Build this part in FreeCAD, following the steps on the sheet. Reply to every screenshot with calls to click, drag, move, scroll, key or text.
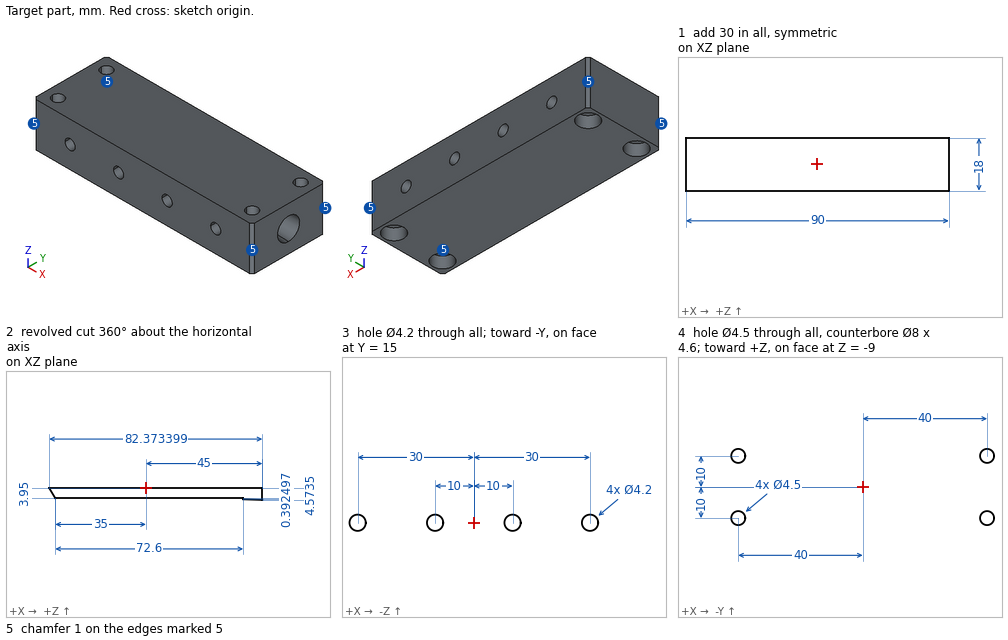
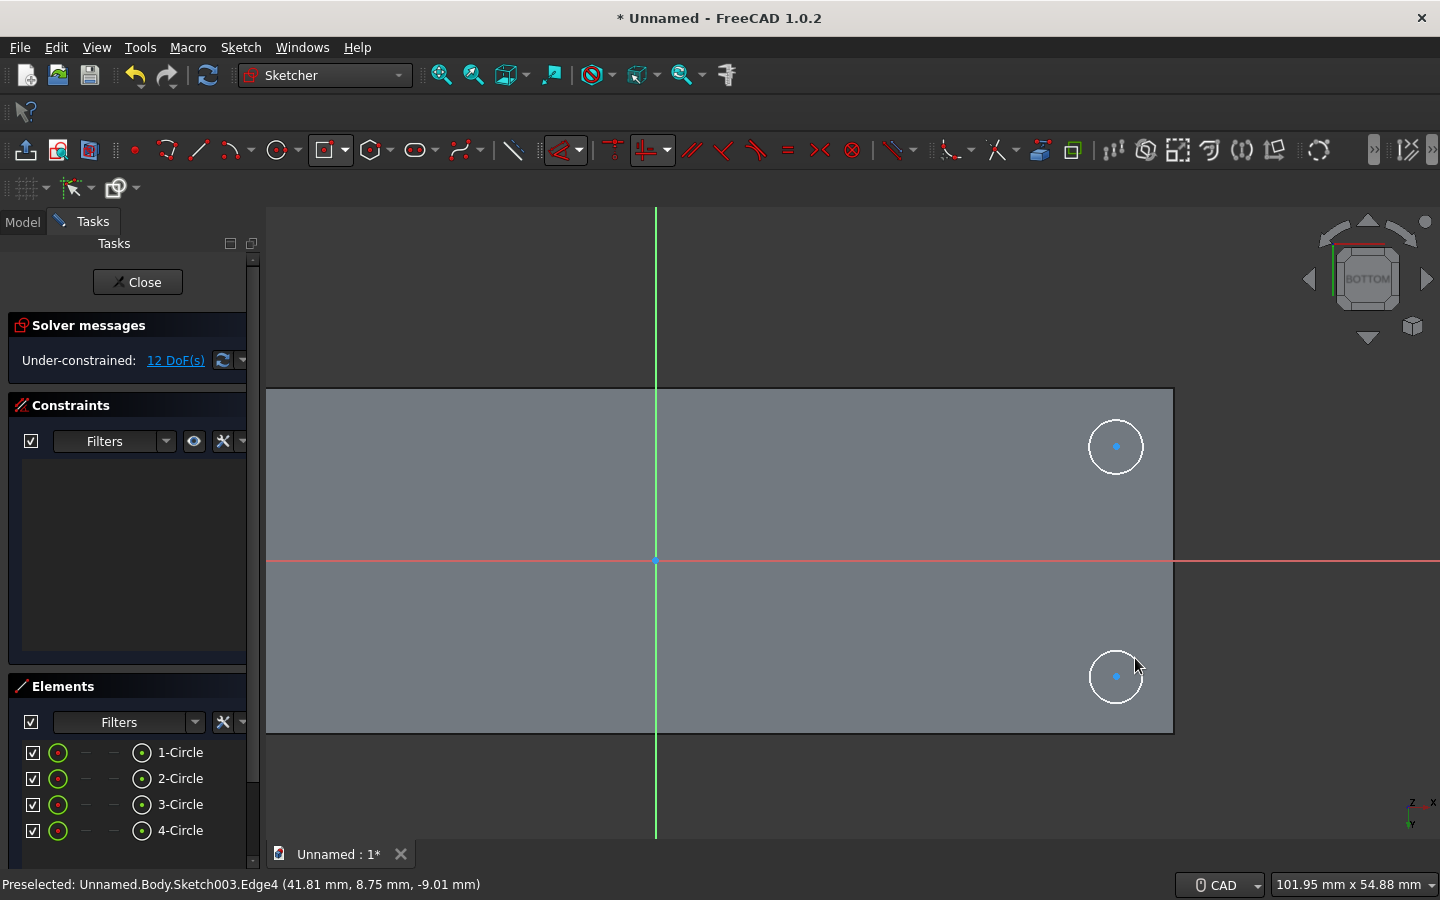
scroll(1046, 446, down, 2)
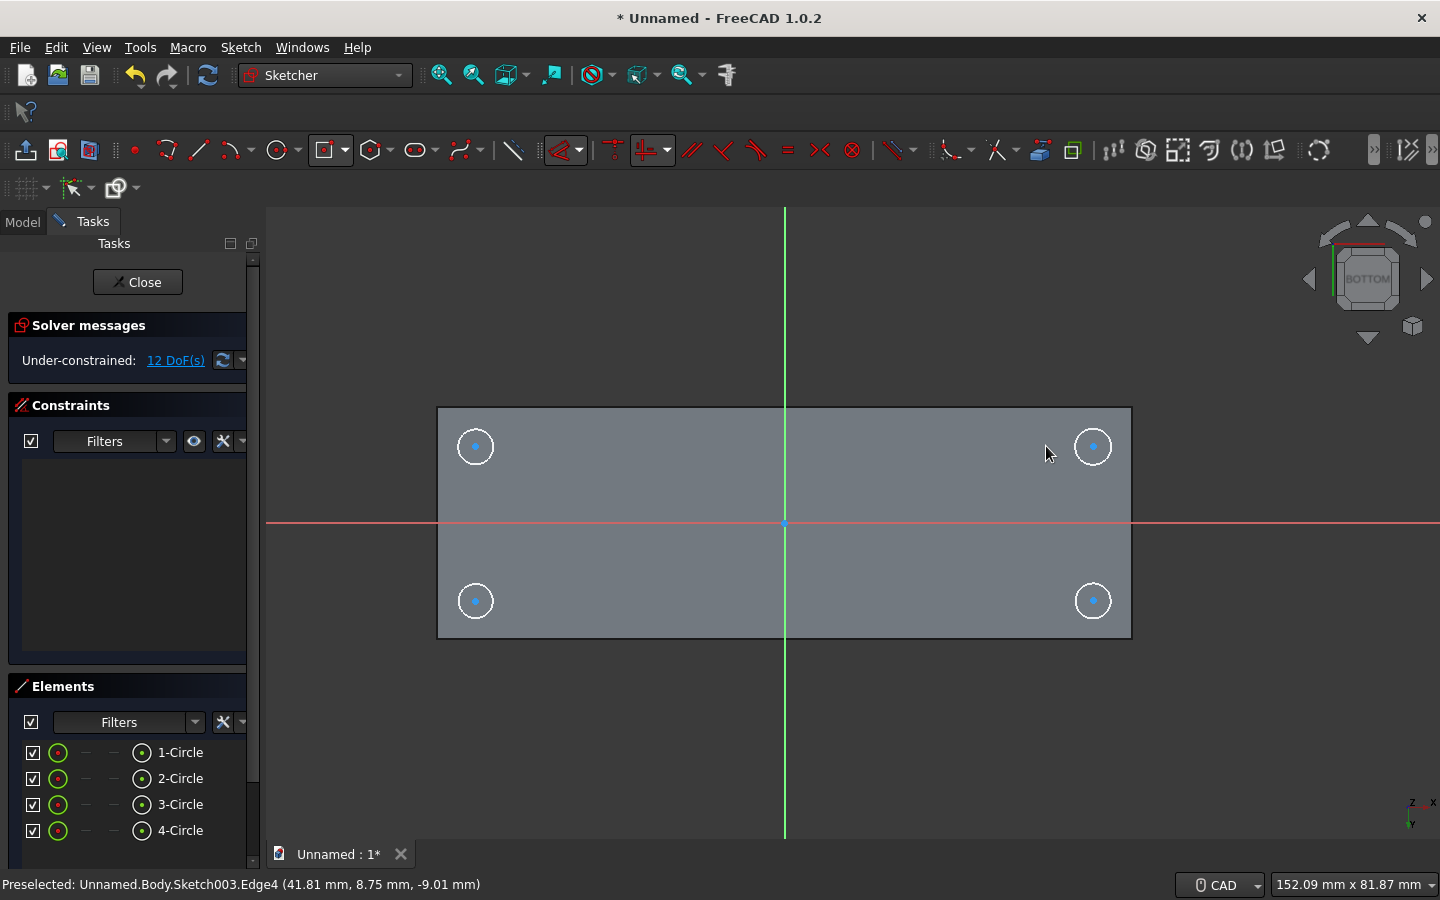
click(488, 589)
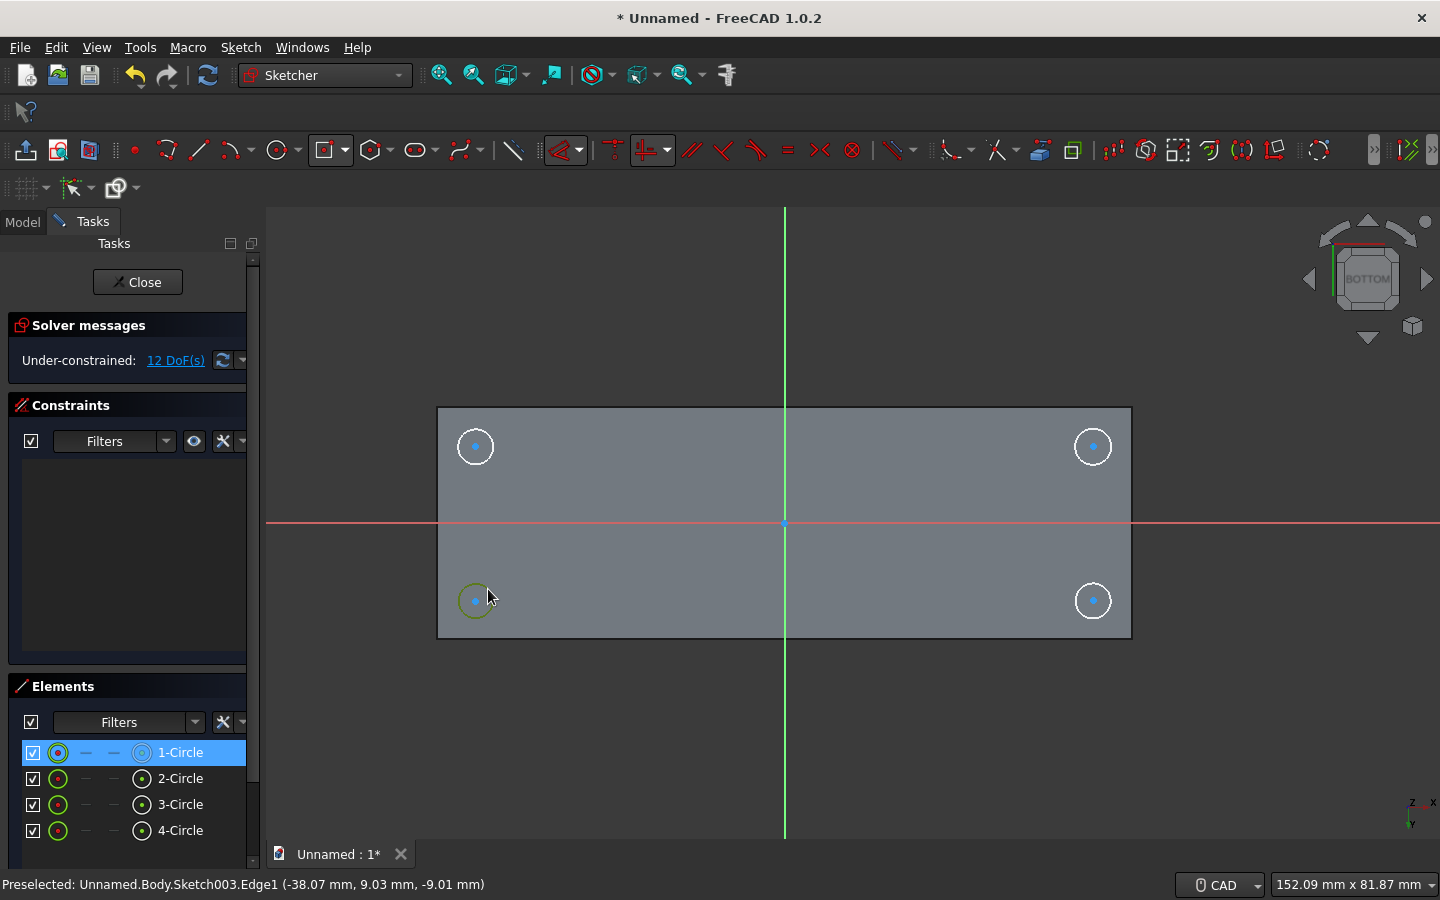
click(488, 434)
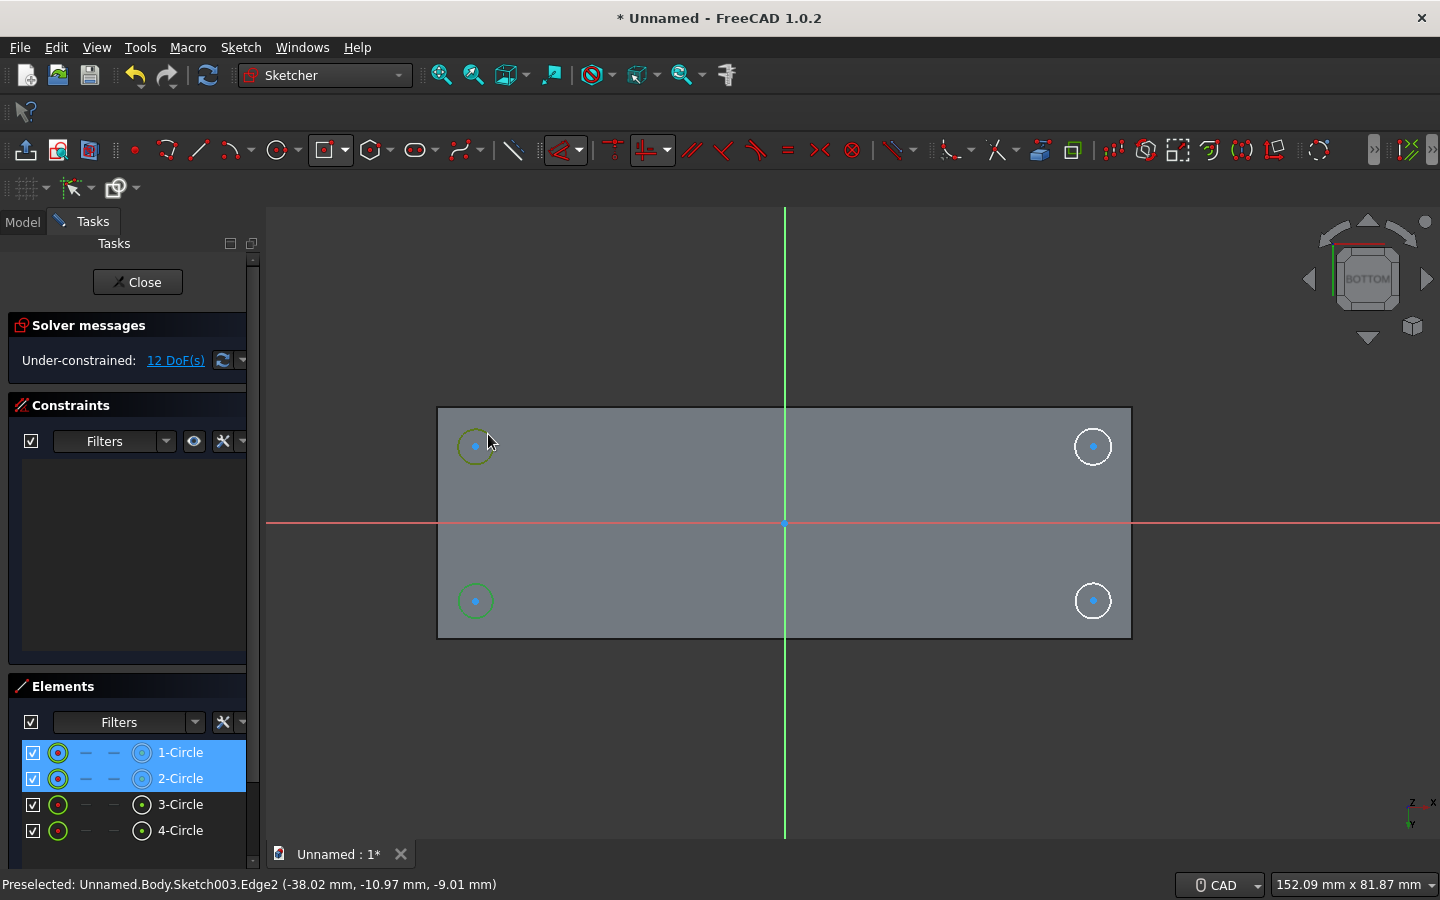
click(1106, 434)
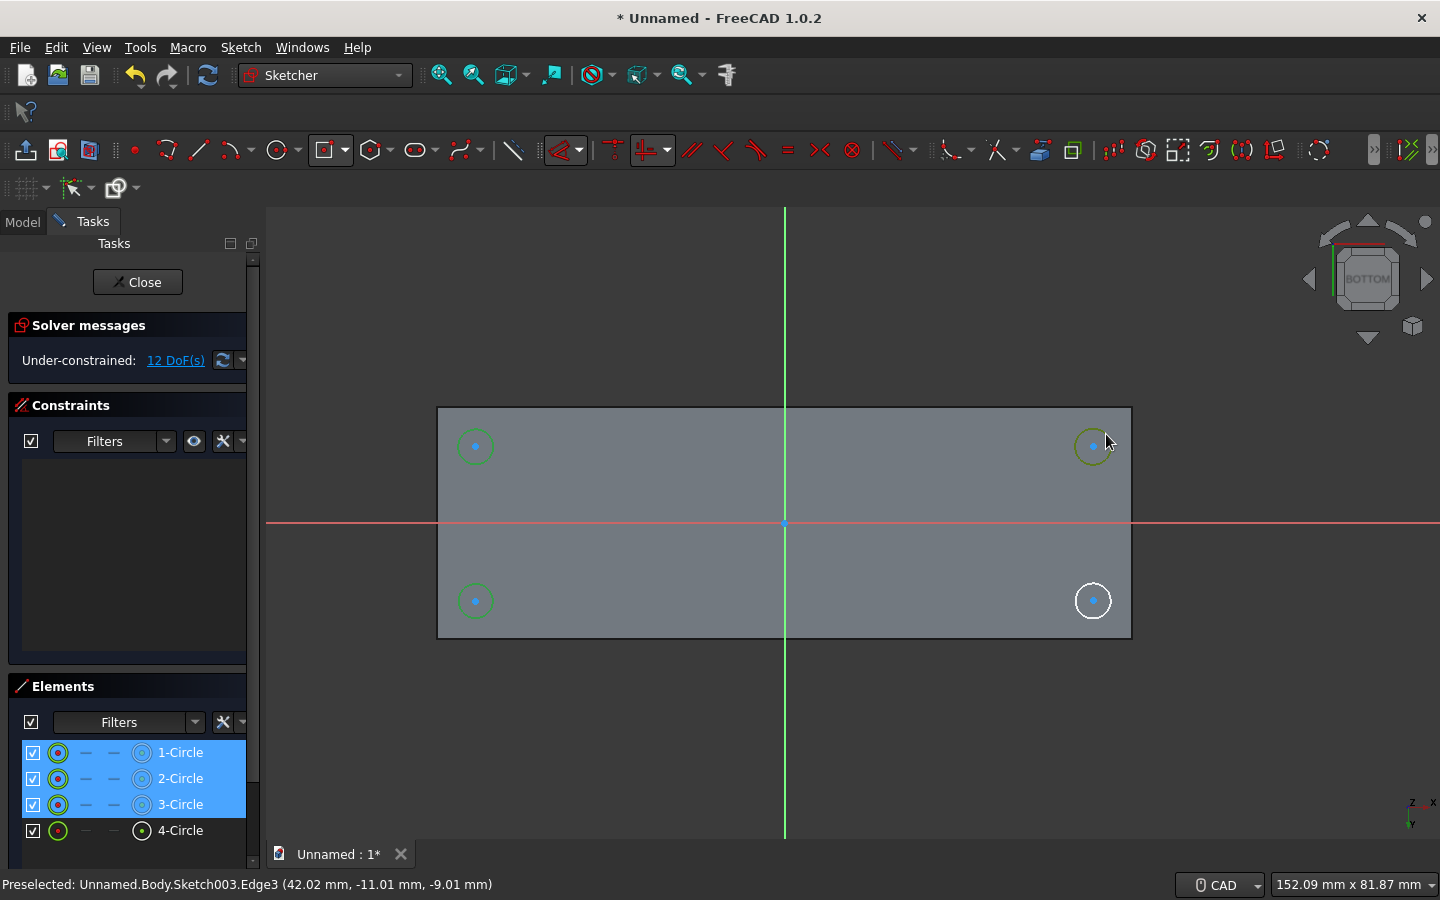
click(1106, 589)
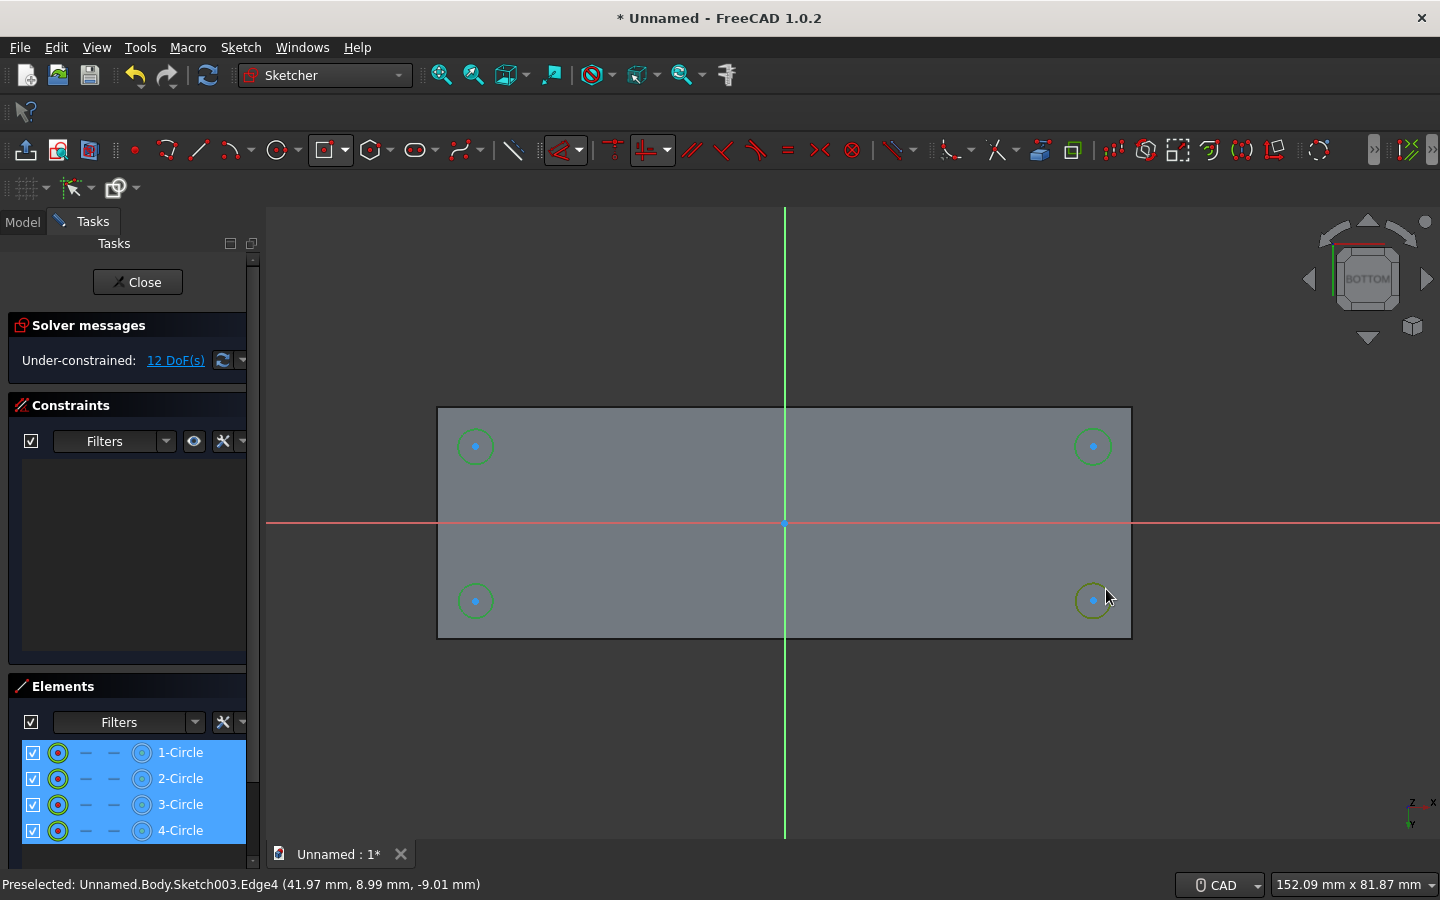
click(788, 150)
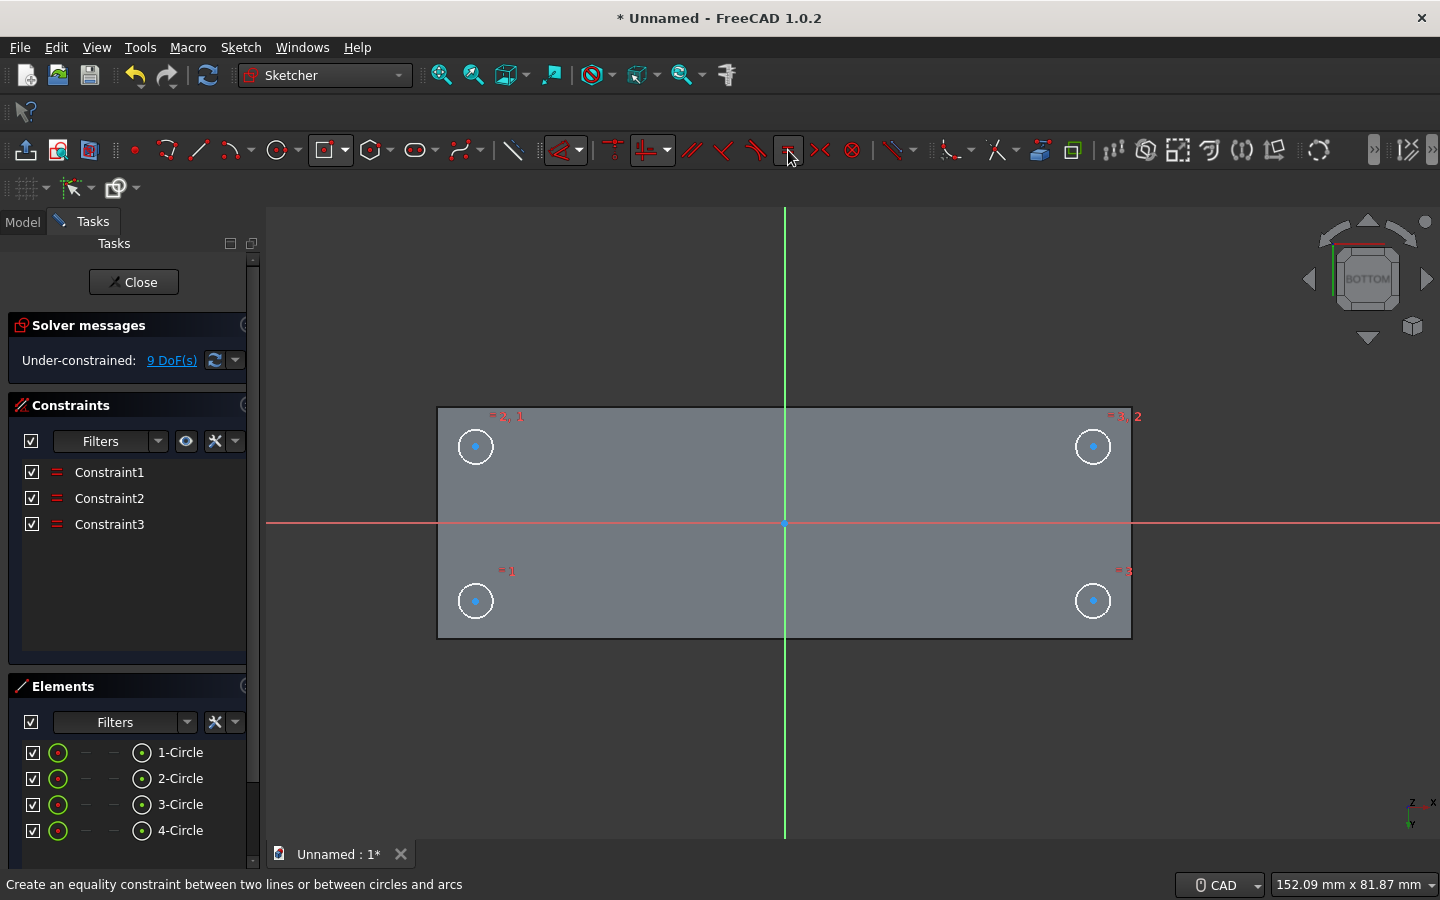
click(476, 601)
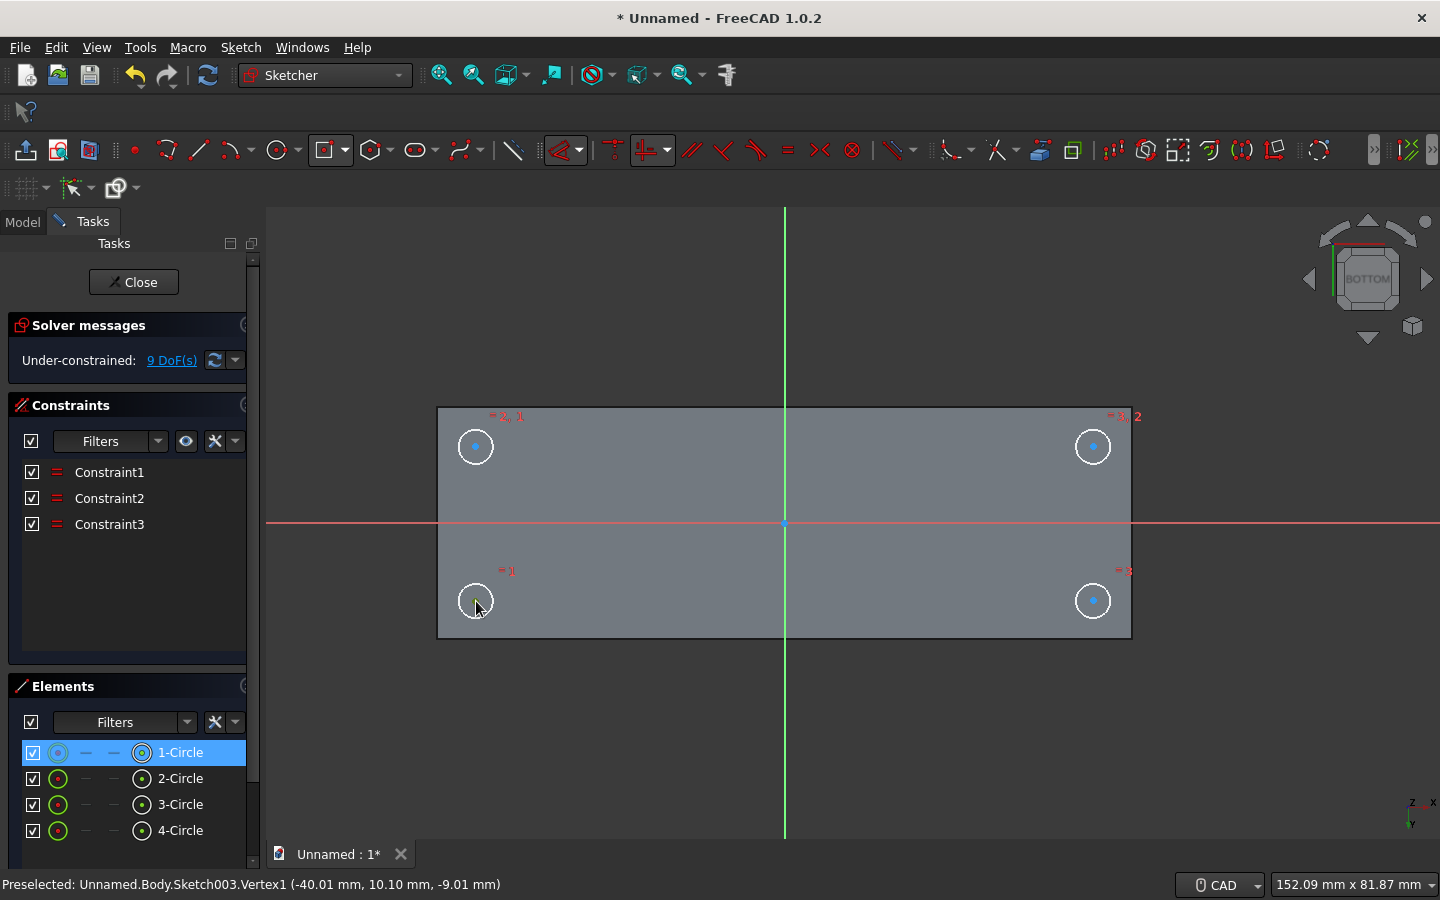
click(476, 447)